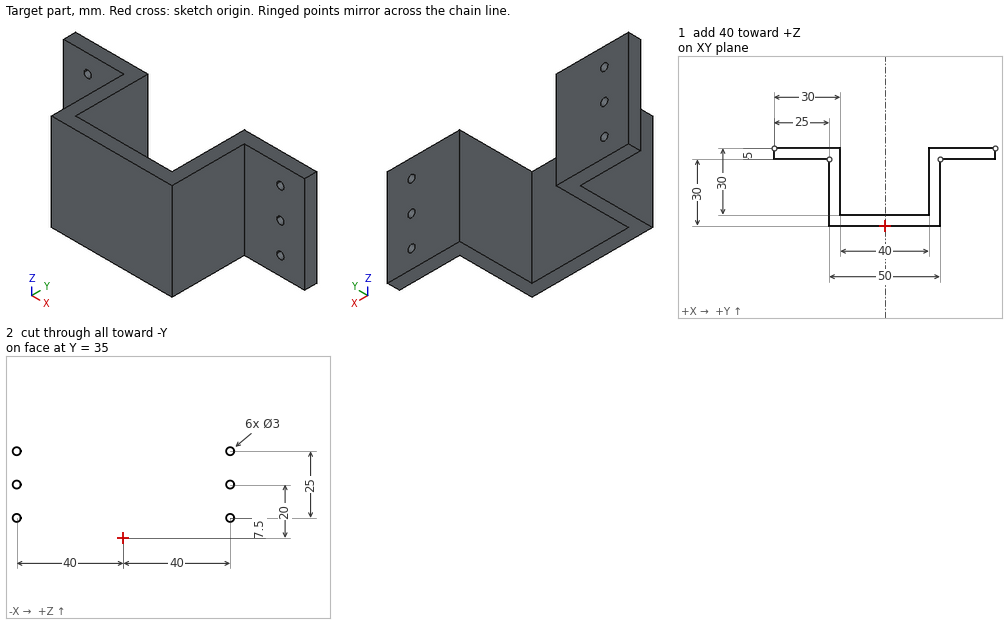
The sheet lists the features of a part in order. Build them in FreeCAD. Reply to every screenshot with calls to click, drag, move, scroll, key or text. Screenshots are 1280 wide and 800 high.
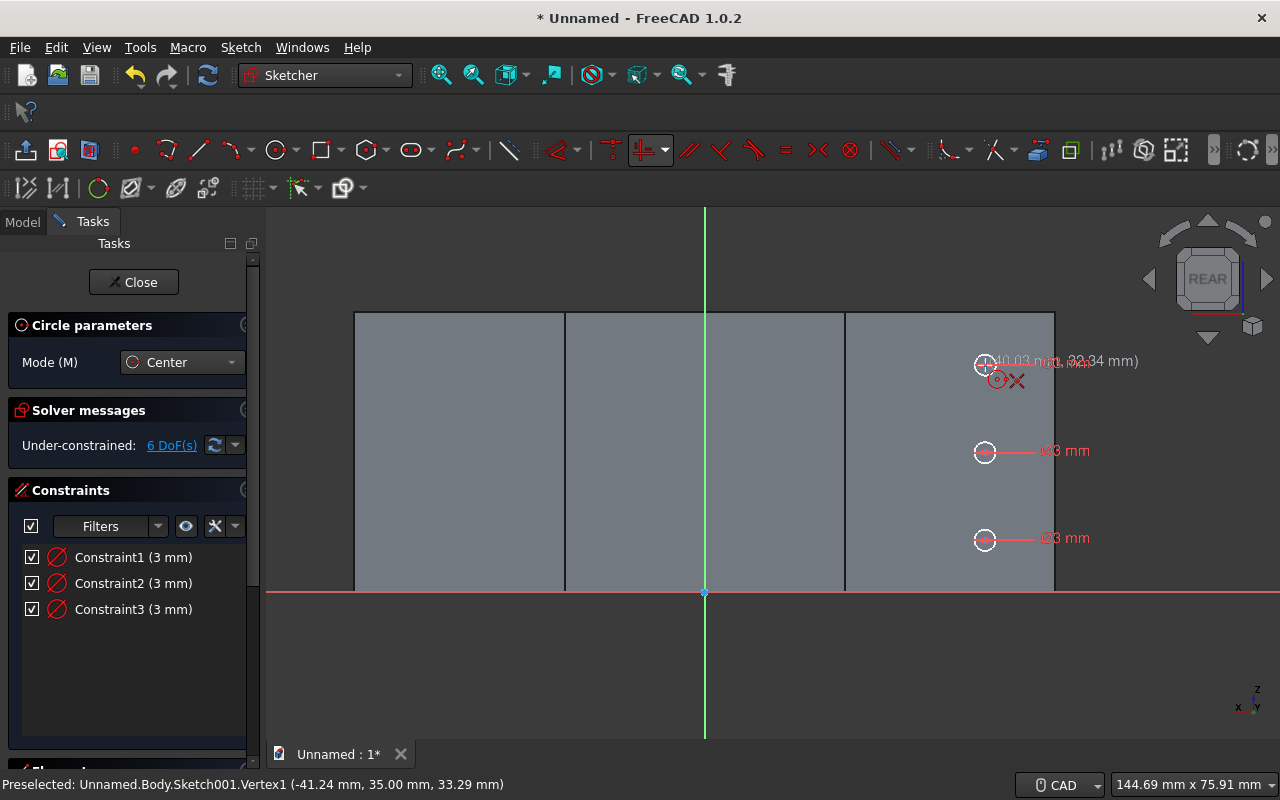
scroll(425, 540, up, 4)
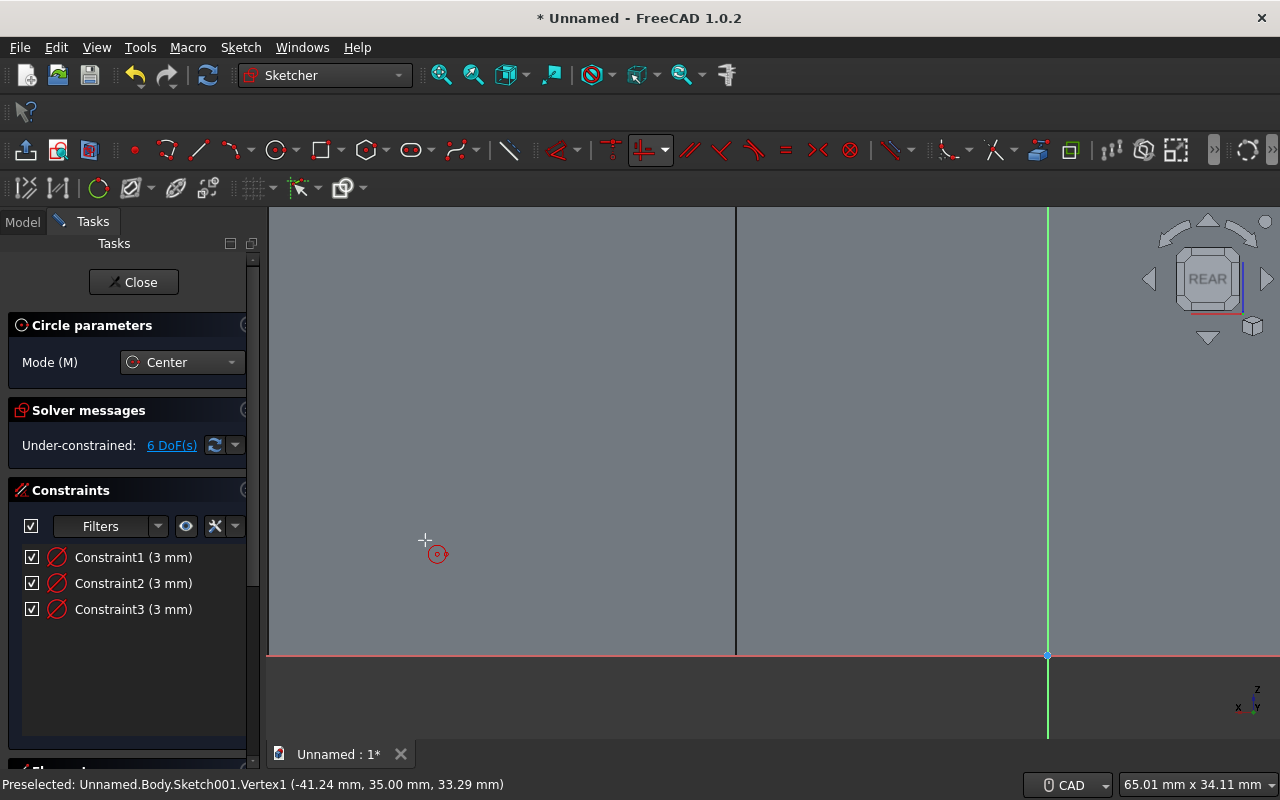
click(424, 539)
move(440, 522)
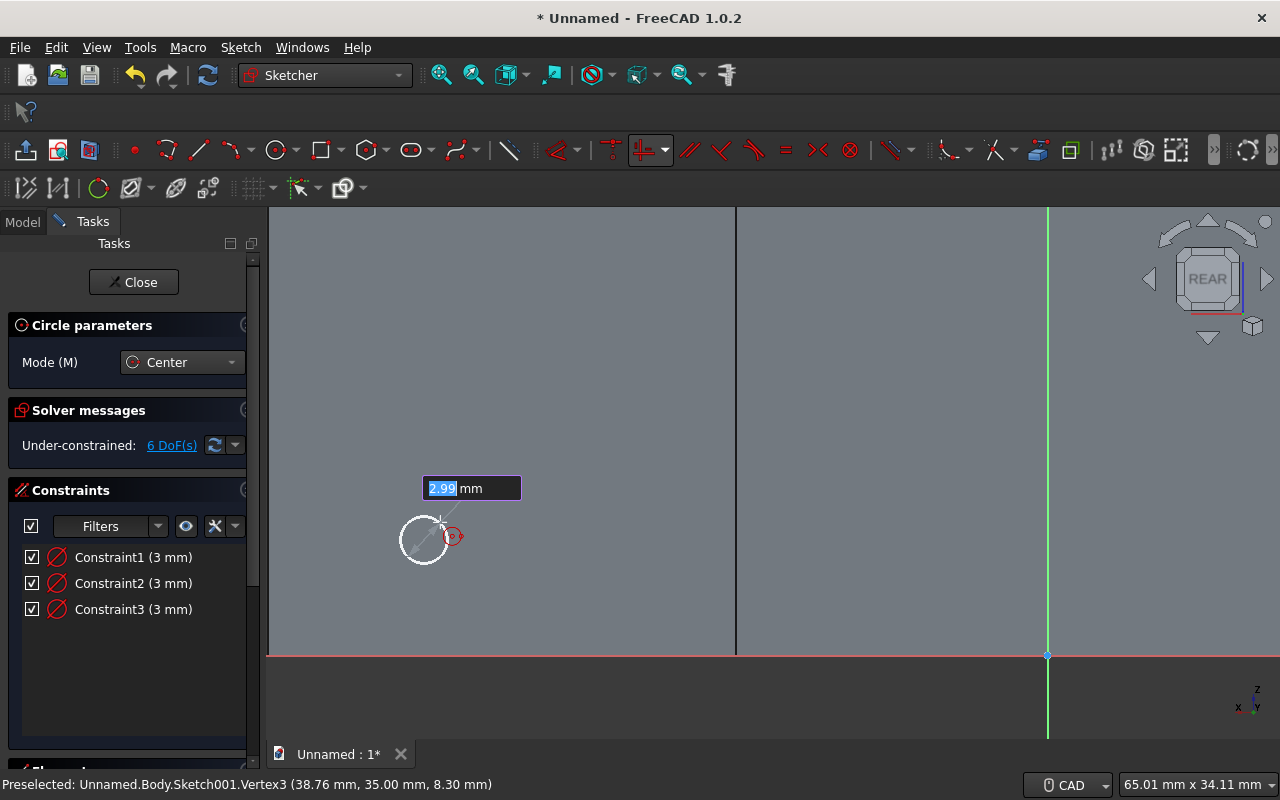
text(3)
key(Return)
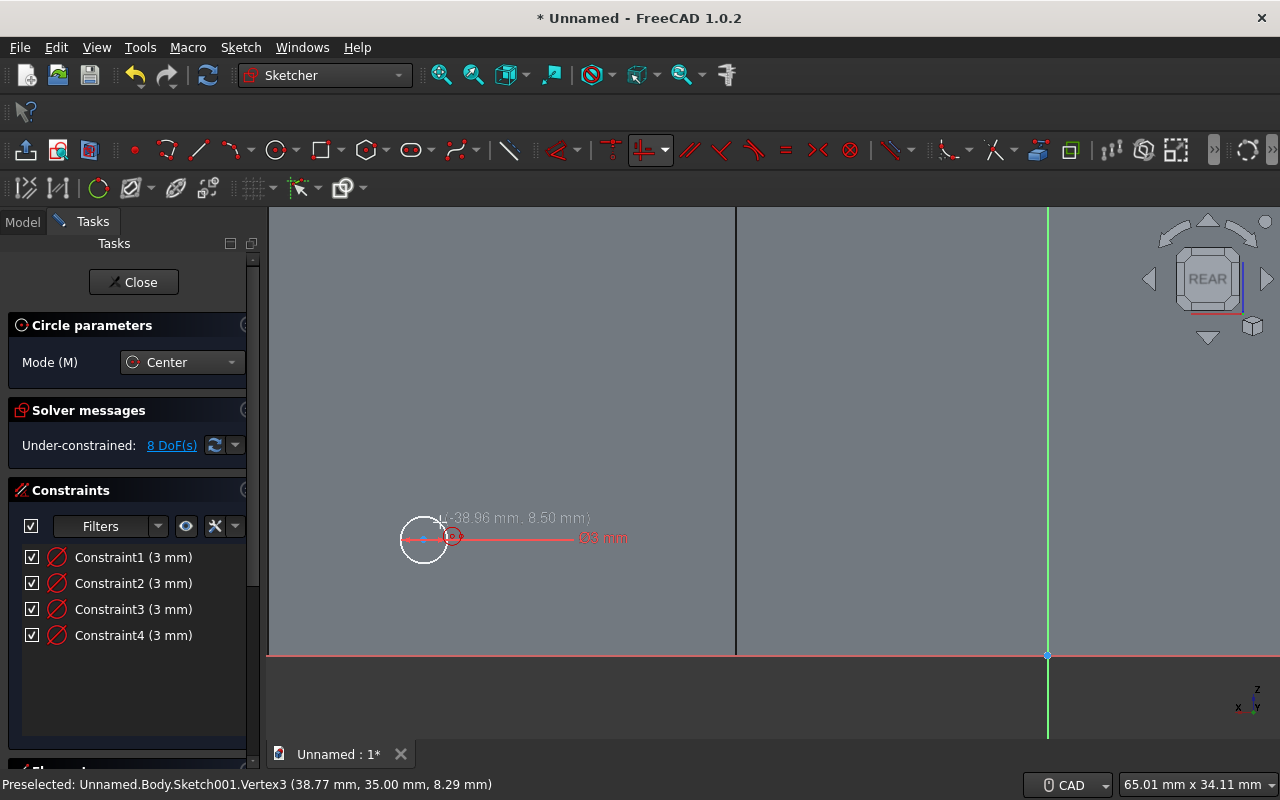
click(424, 344)
move(440, 327)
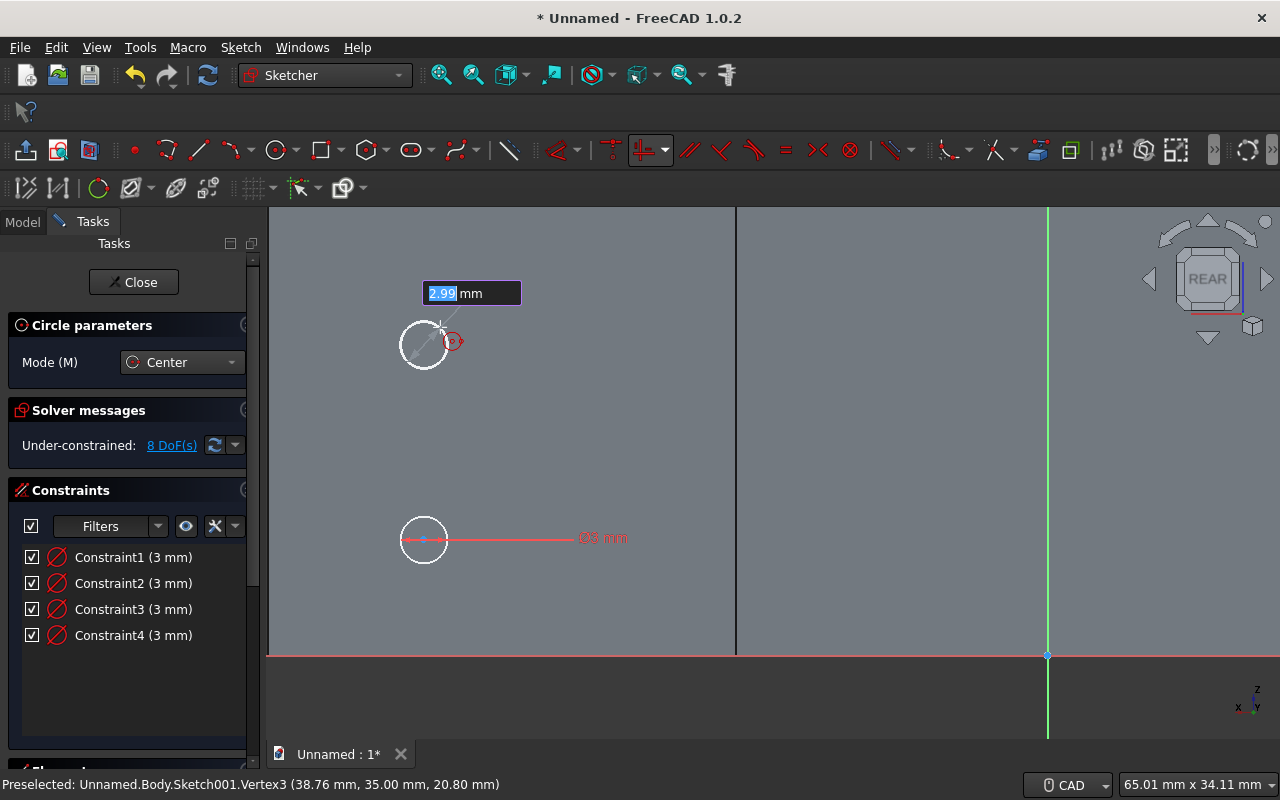
text(3)
key(Return)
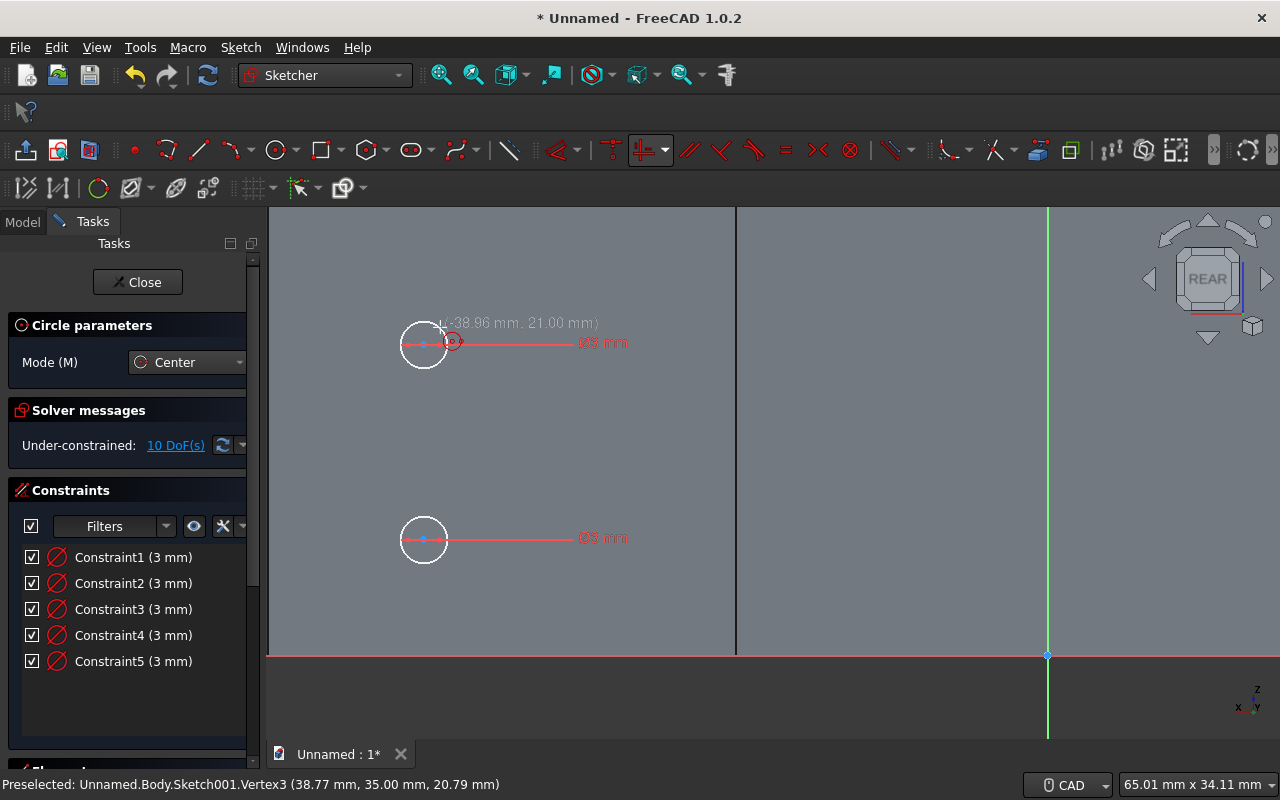
scroll(424, 540, down, 4)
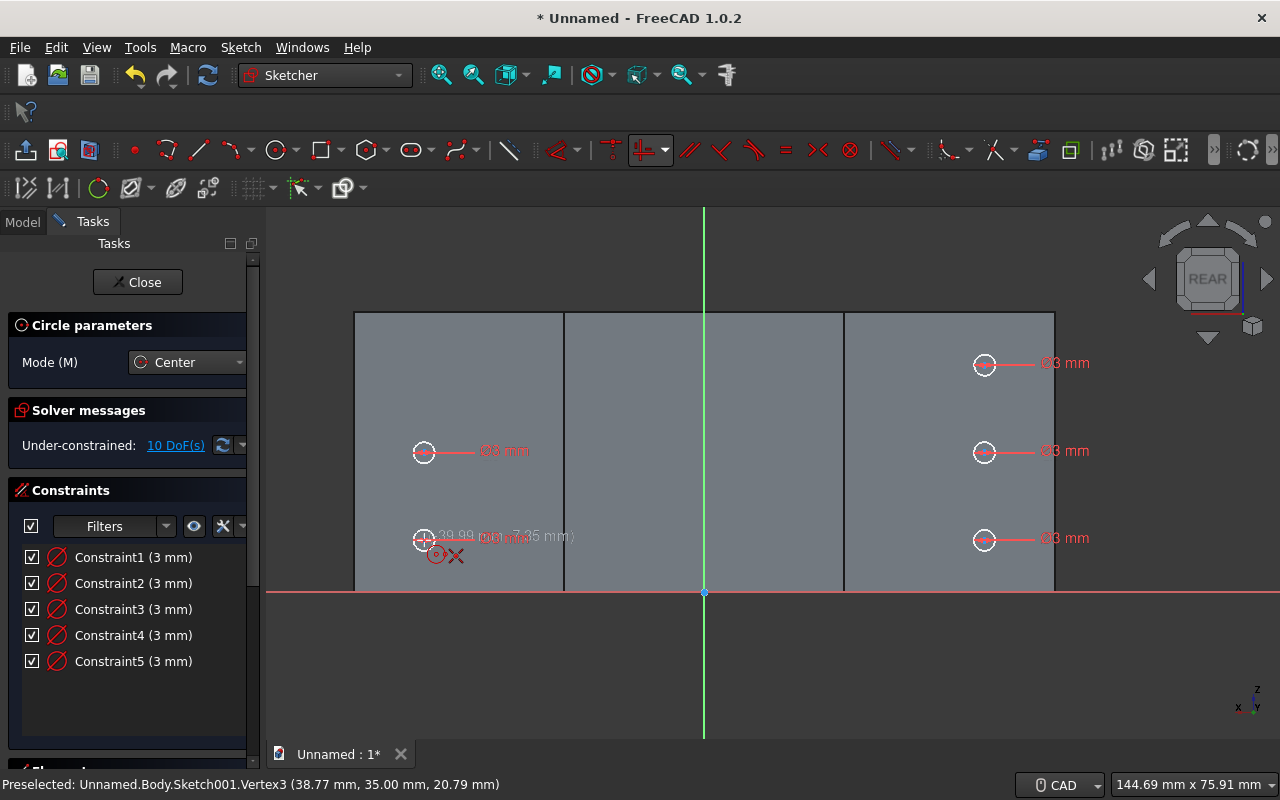
scroll(424, 365, up, 4)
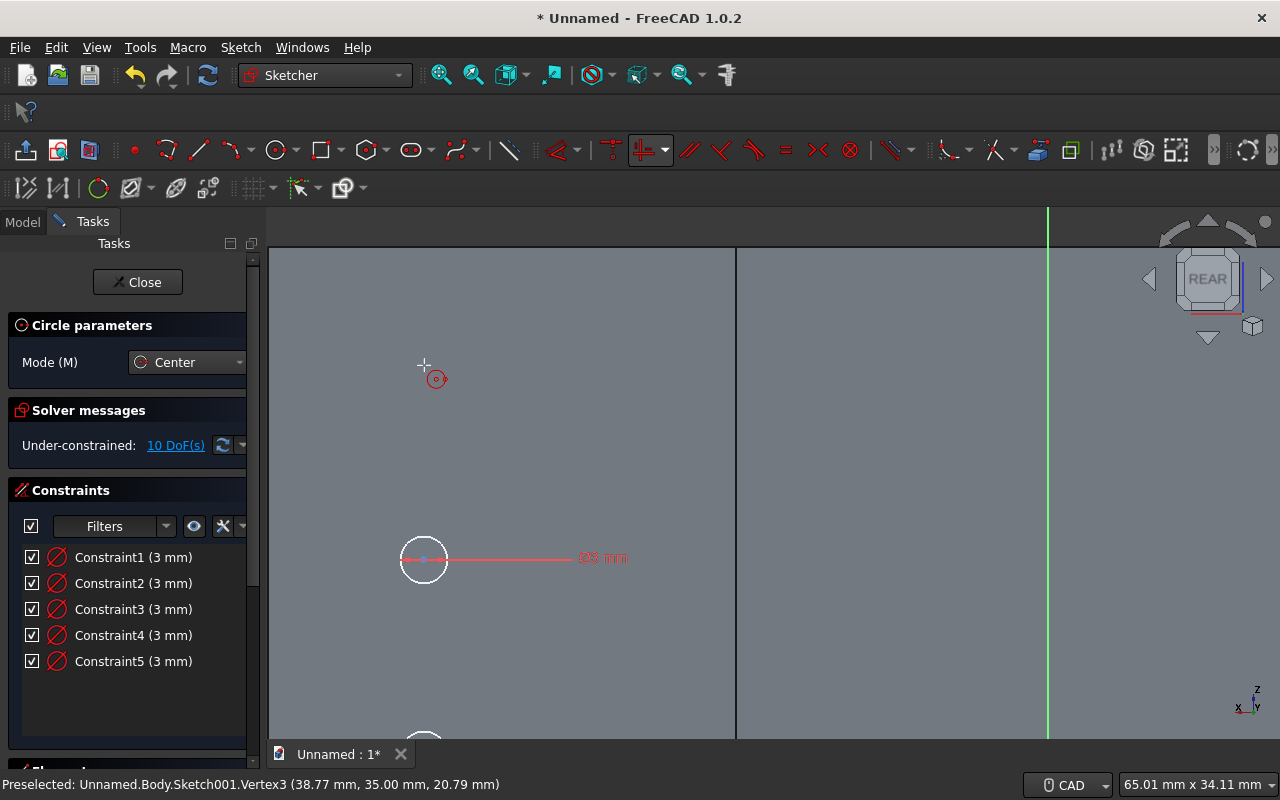
click(424, 364)
move(440, 347)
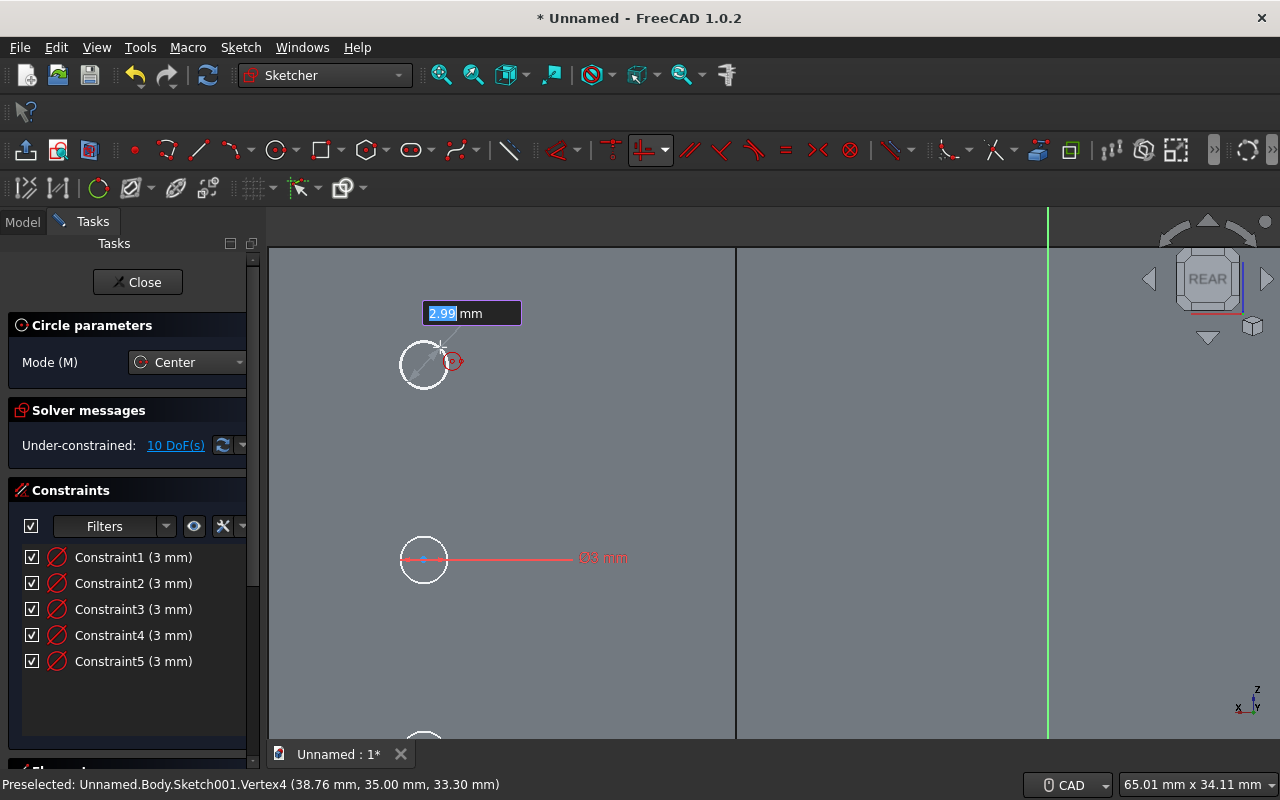
text(3)
key(Return)
key(Escape)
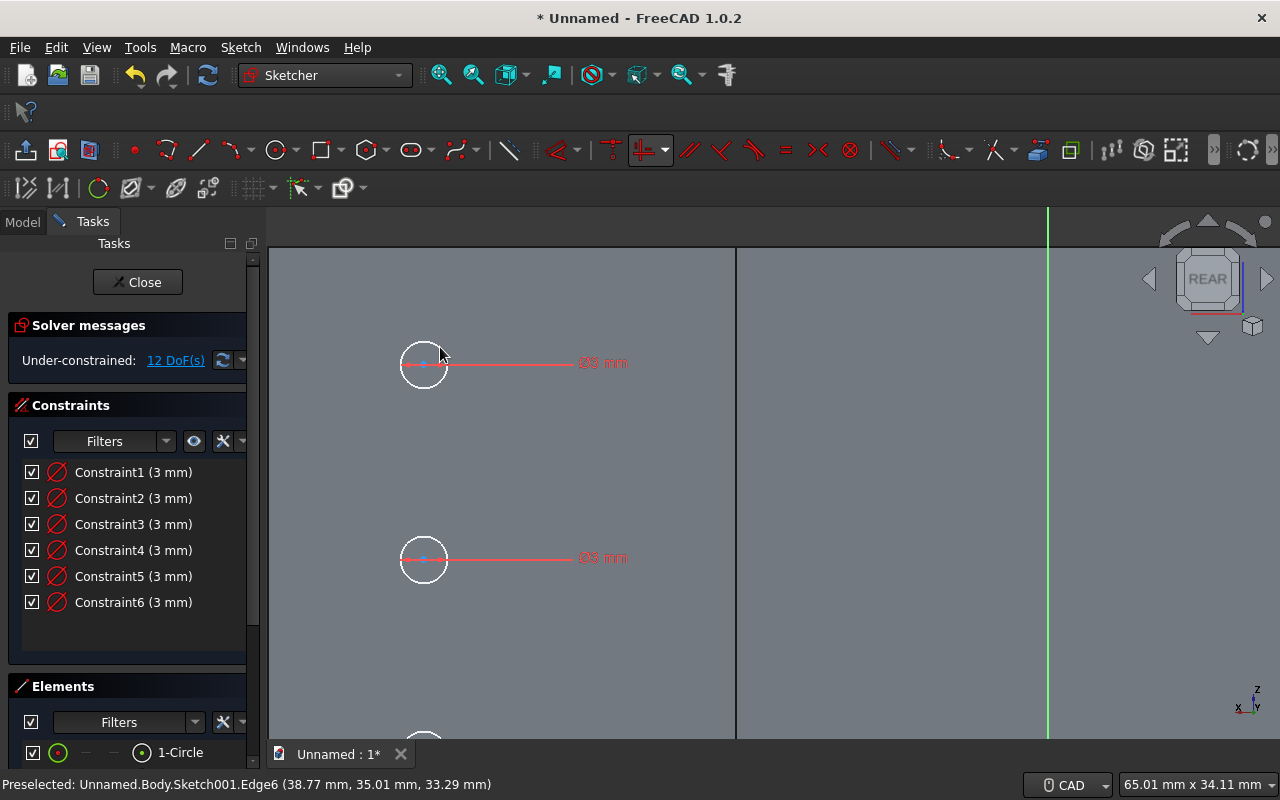
scroll(424, 365, down, 4)